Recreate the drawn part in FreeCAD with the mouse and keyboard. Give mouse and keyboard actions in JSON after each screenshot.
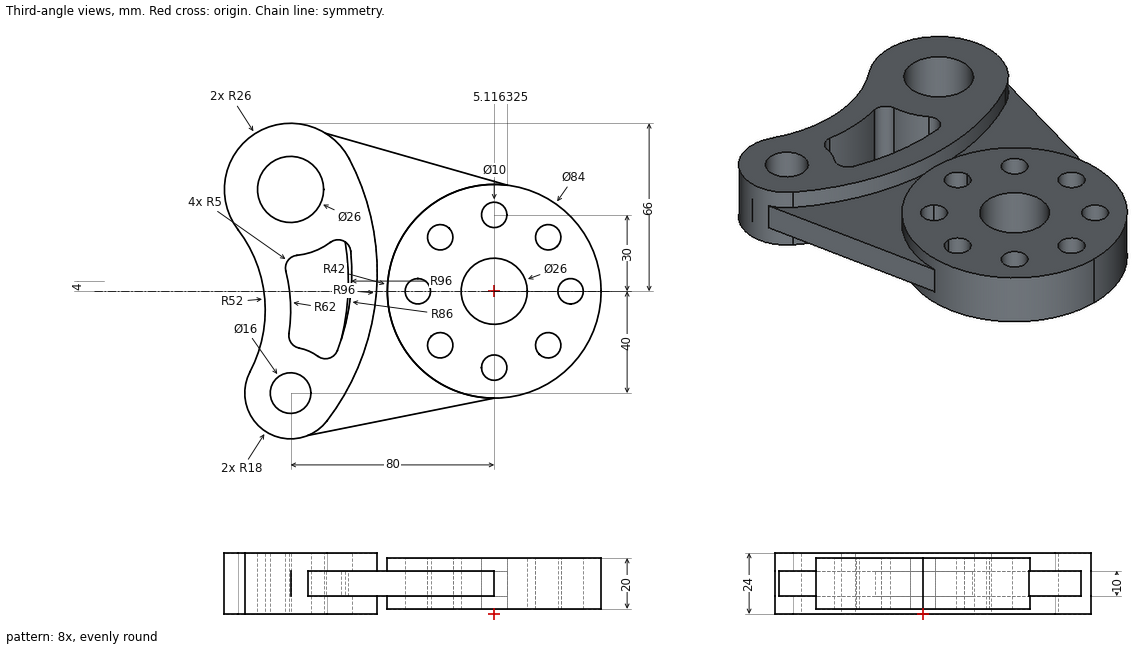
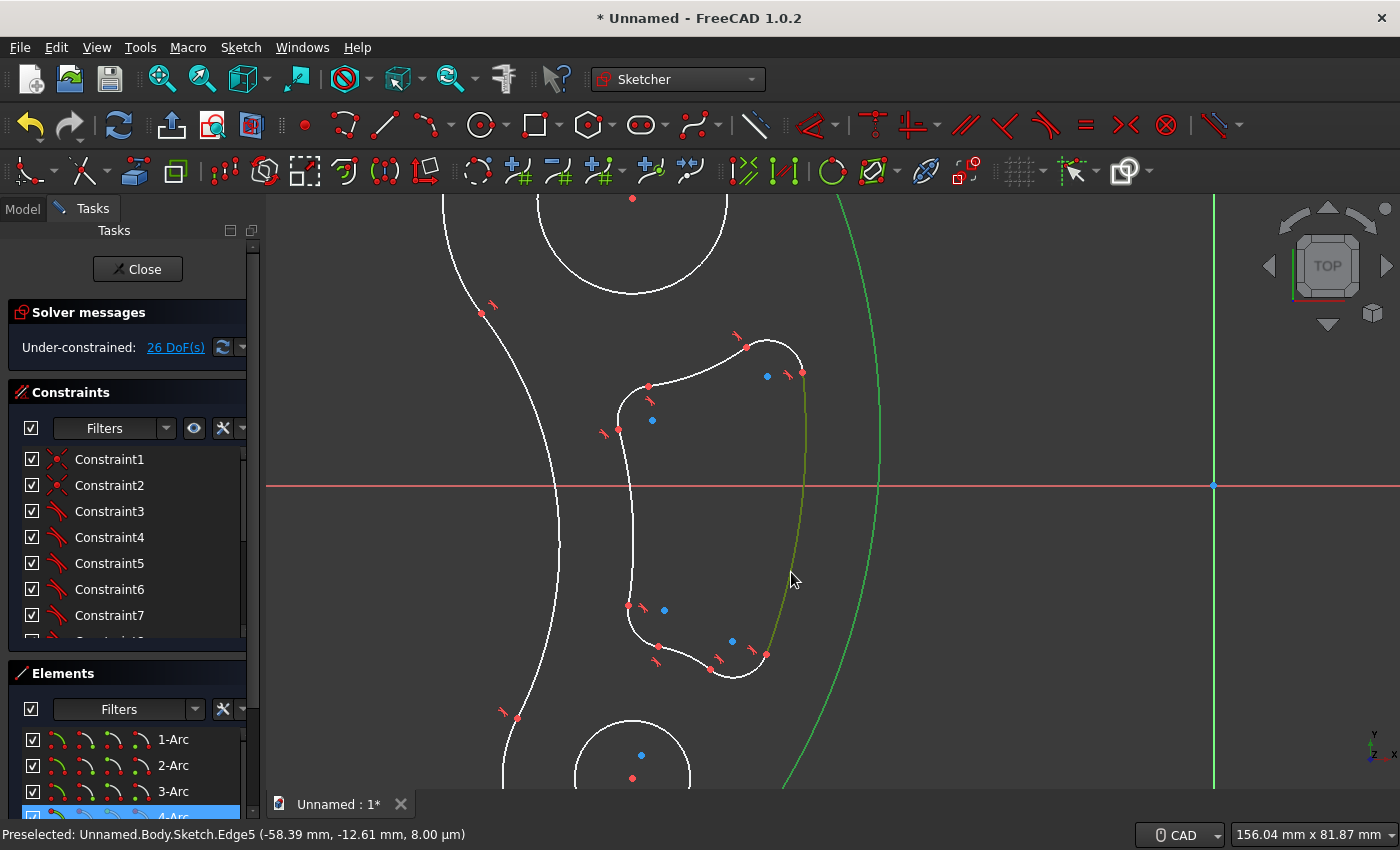
{"action": "left_click", "coordinate": [874, 126]}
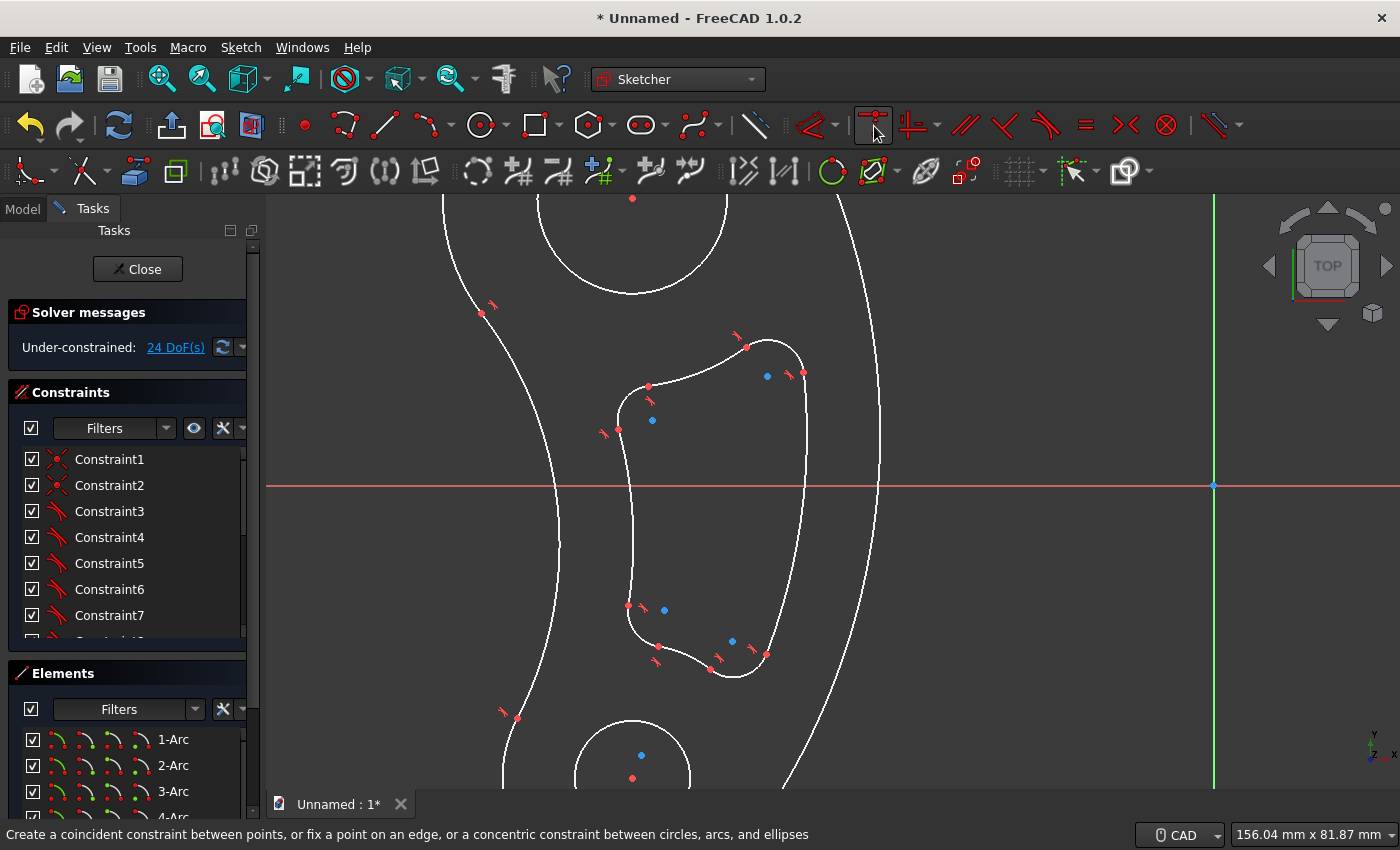
{"action": "left_click", "coordinate": [673, 738]}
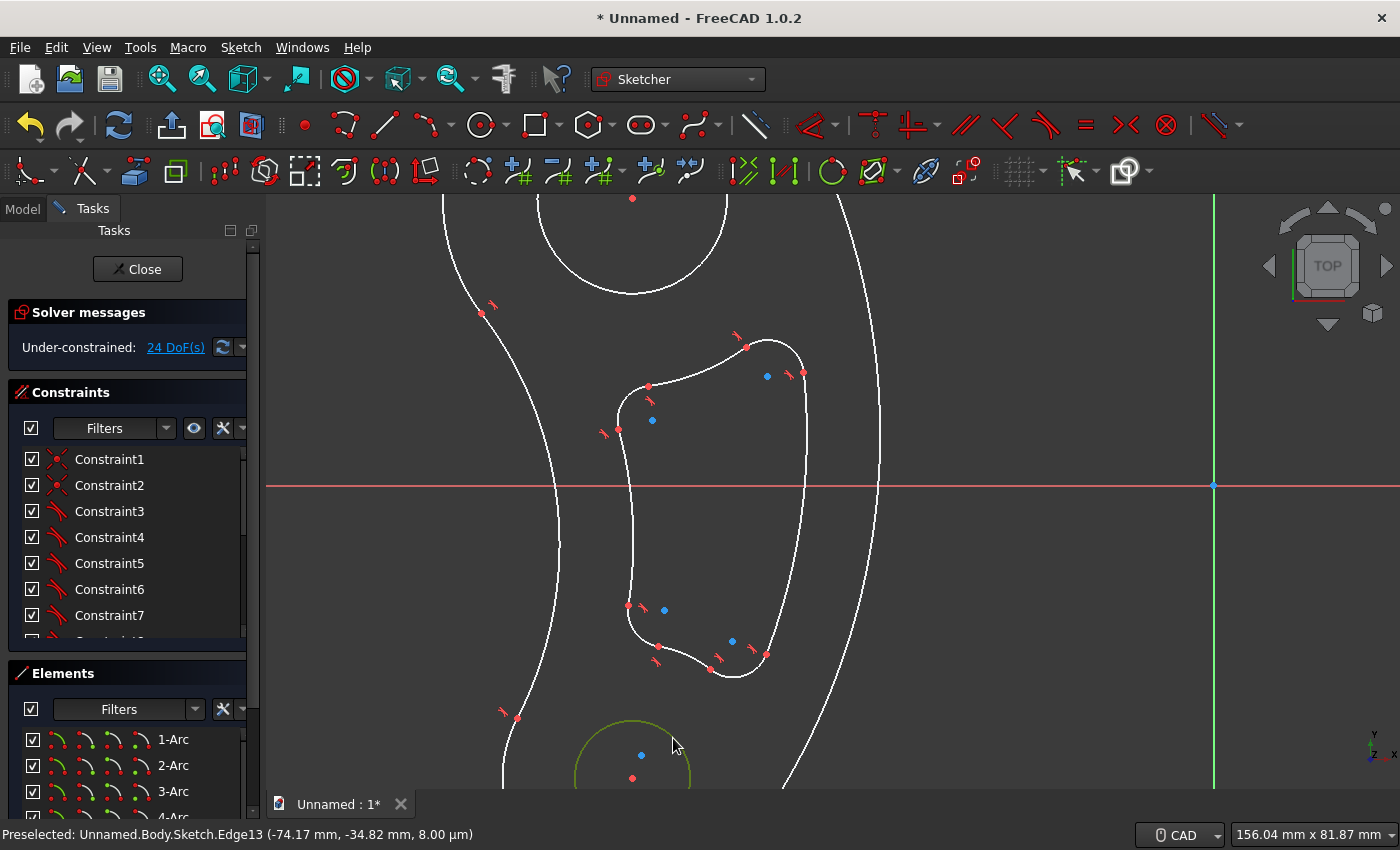
{"action": "left_click", "coordinate": [696, 660]}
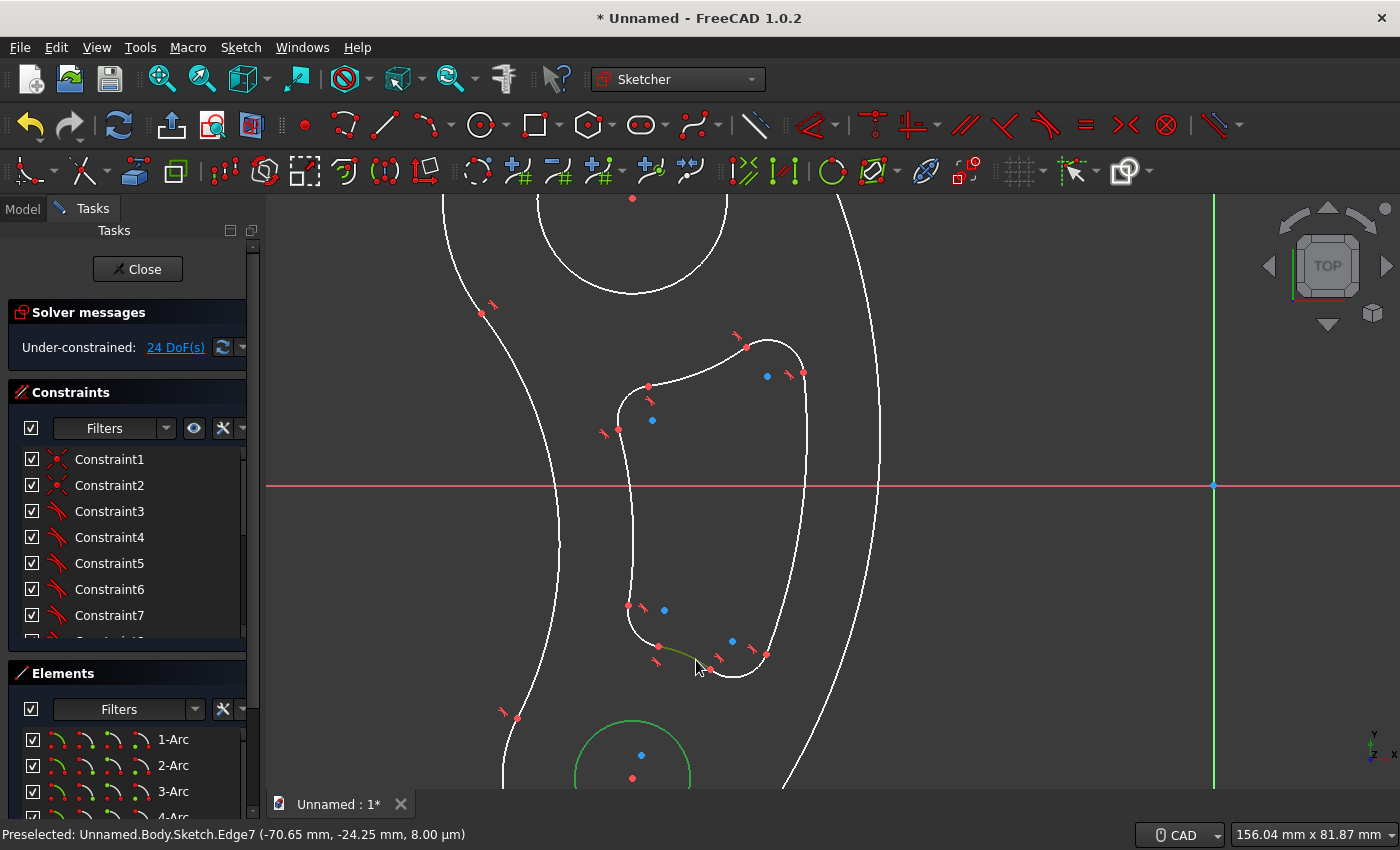
{"action": "left_click", "coordinate": [874, 126]}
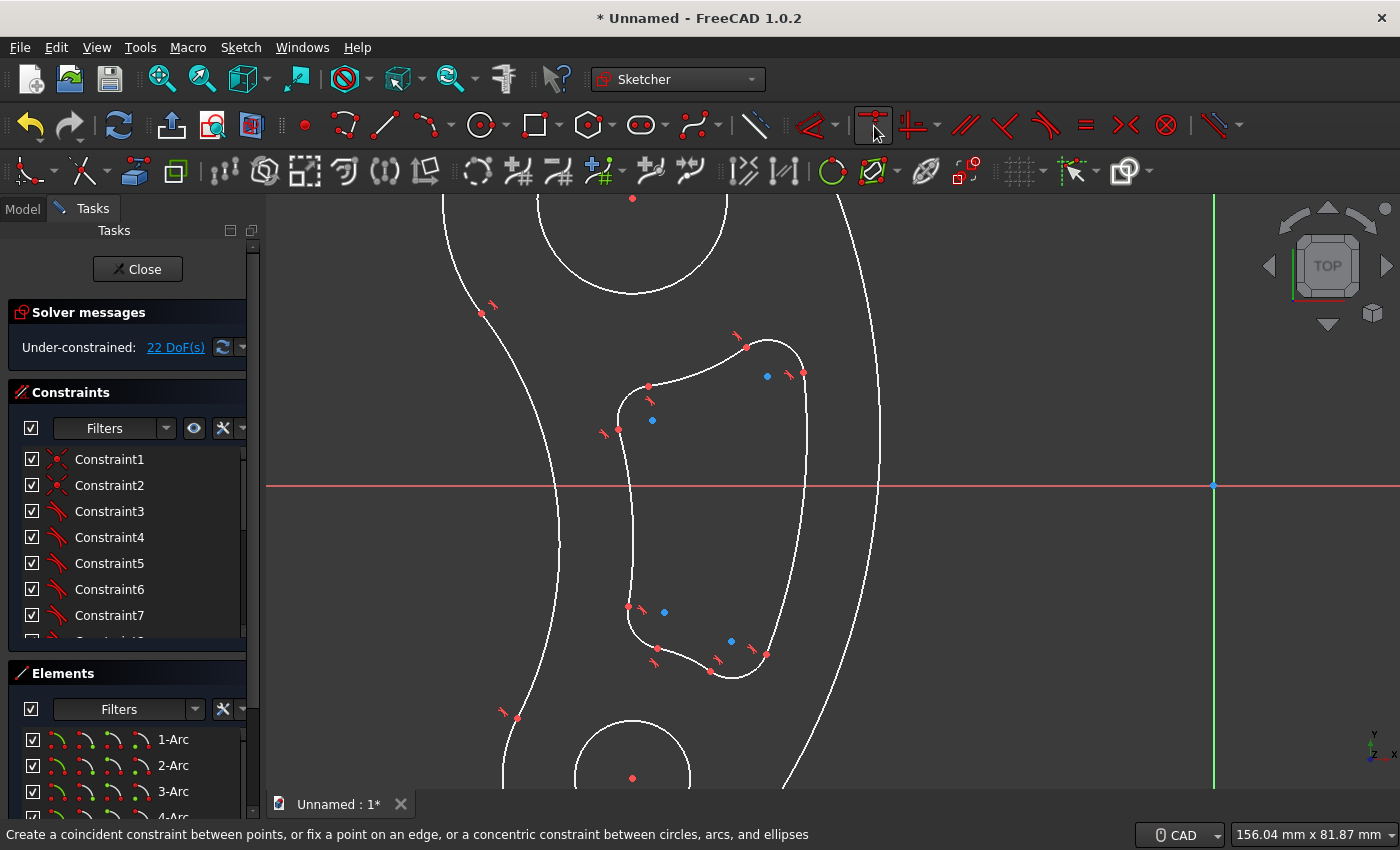
{"action": "left_click", "coordinate": [556, 597]}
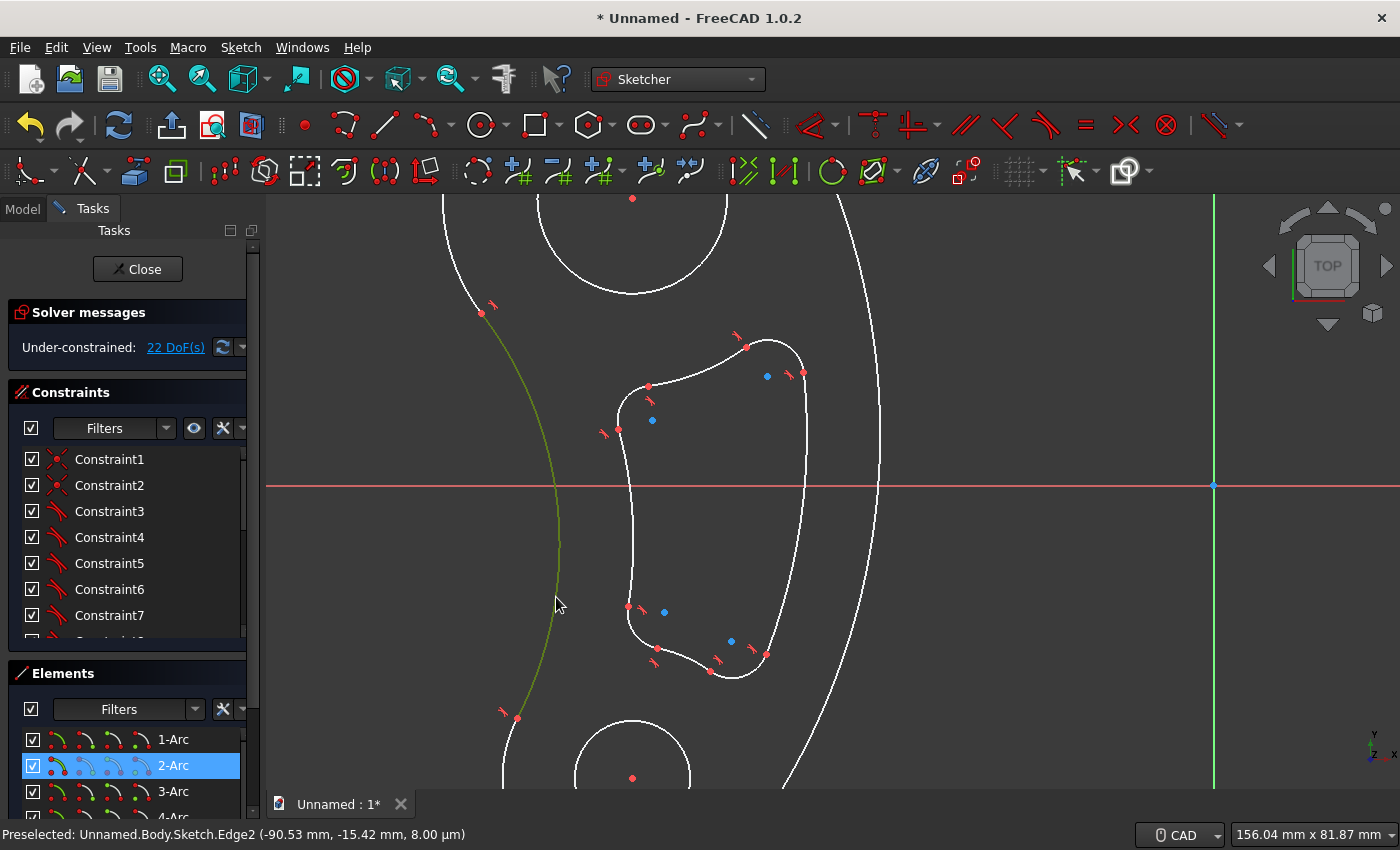
{"action": "left_click", "coordinate": [633, 554]}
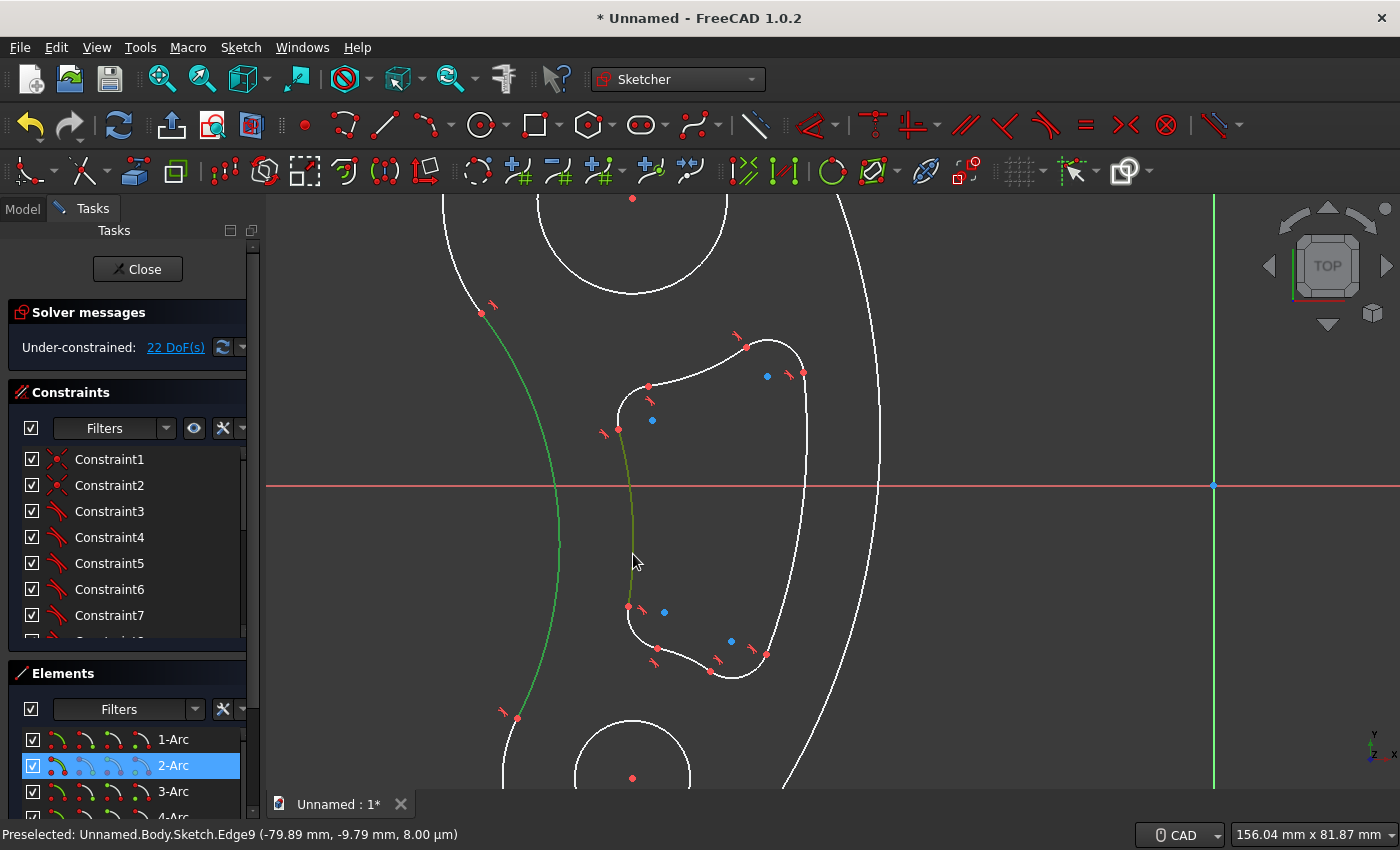
{"action": "left_click", "coordinate": [874, 126]}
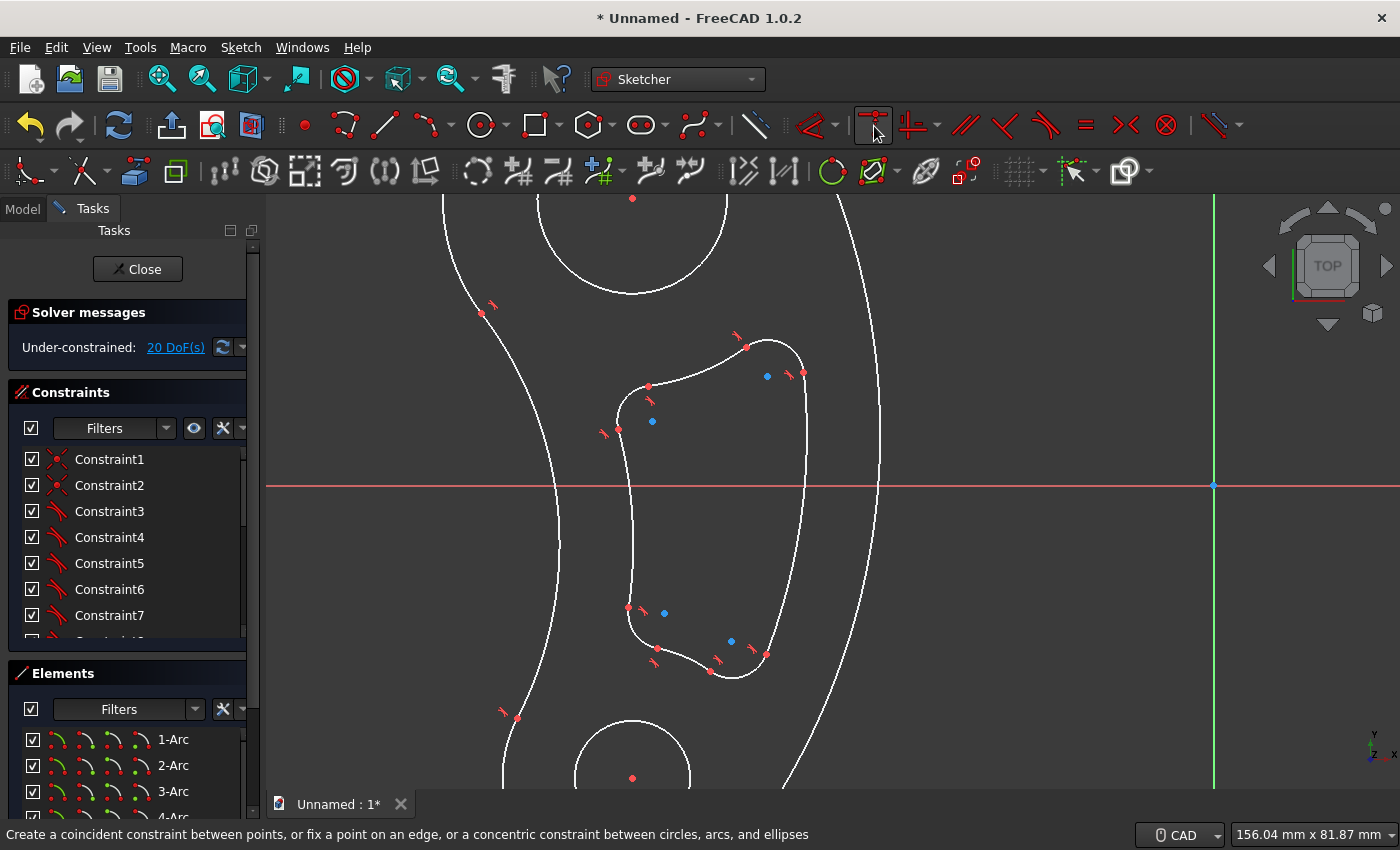
{"action": "left_click", "coordinate": [565, 266]}